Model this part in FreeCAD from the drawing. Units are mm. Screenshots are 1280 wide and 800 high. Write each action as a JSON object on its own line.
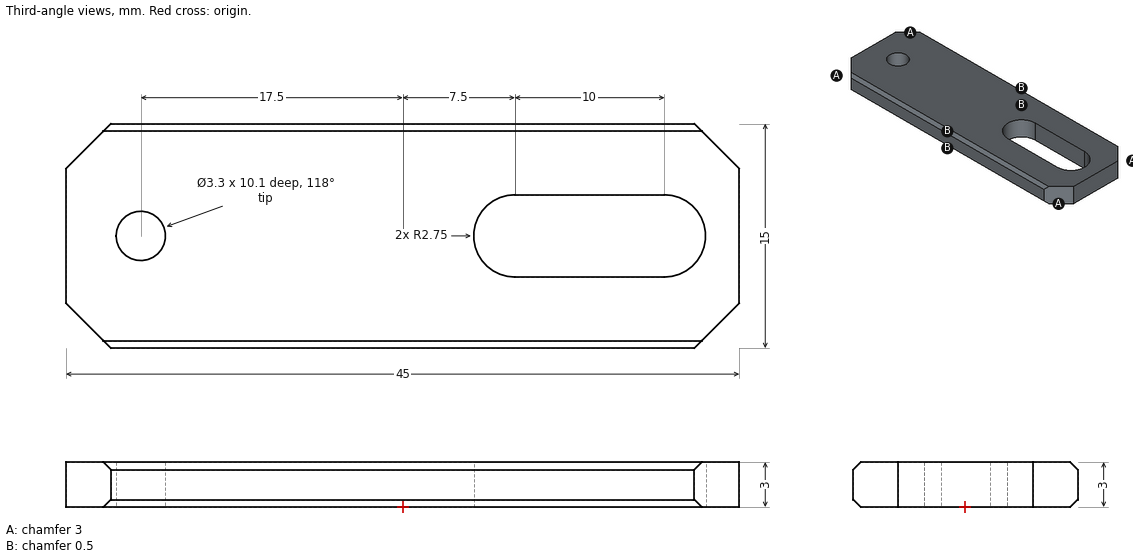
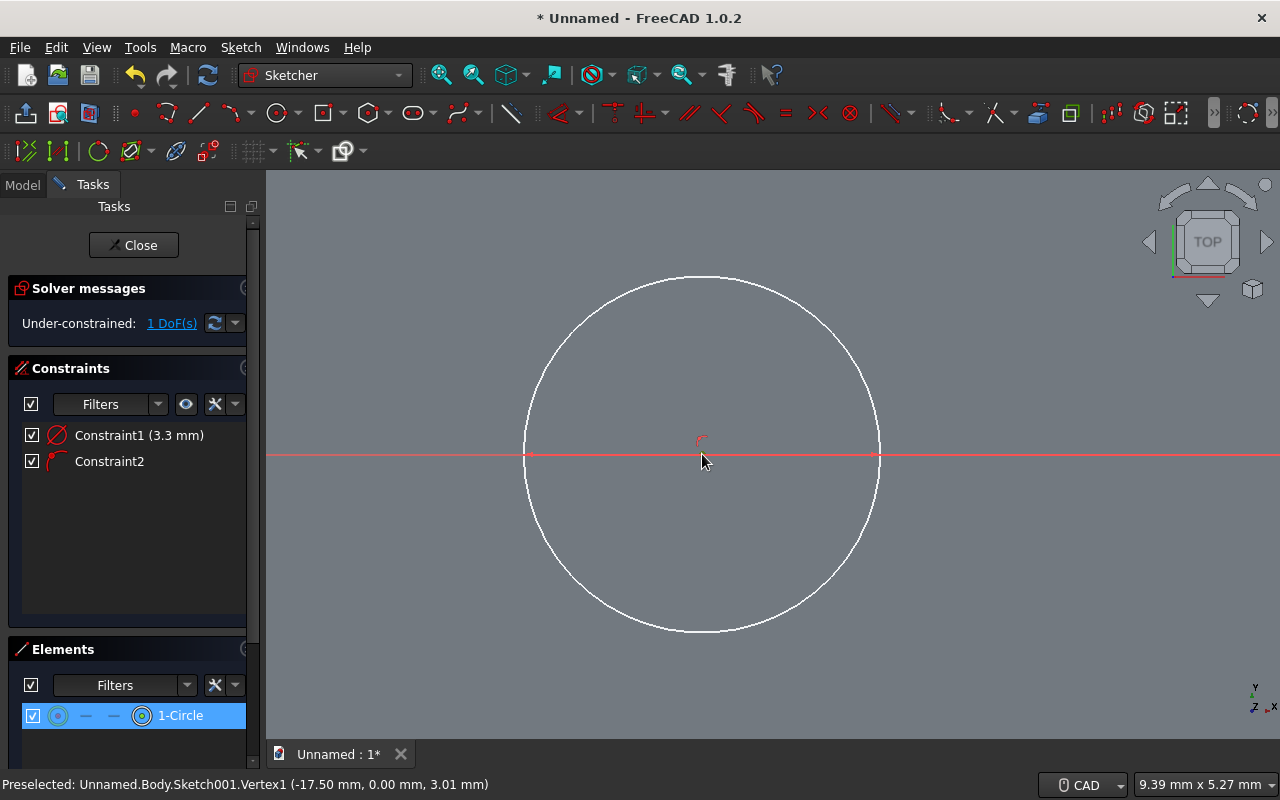
{"action": "key", "text": "l"}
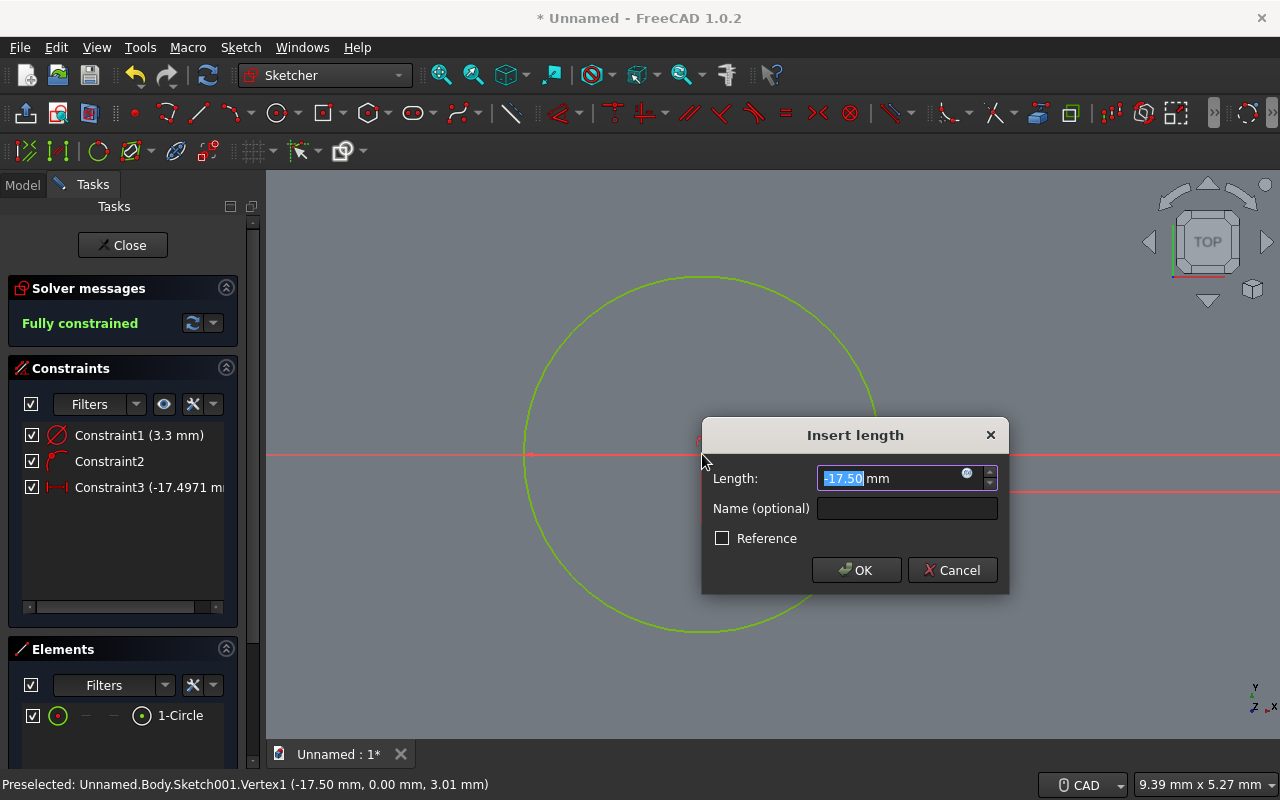
{"action": "type", "text": "-17.5"}
{"action": "key", "text": "Return"}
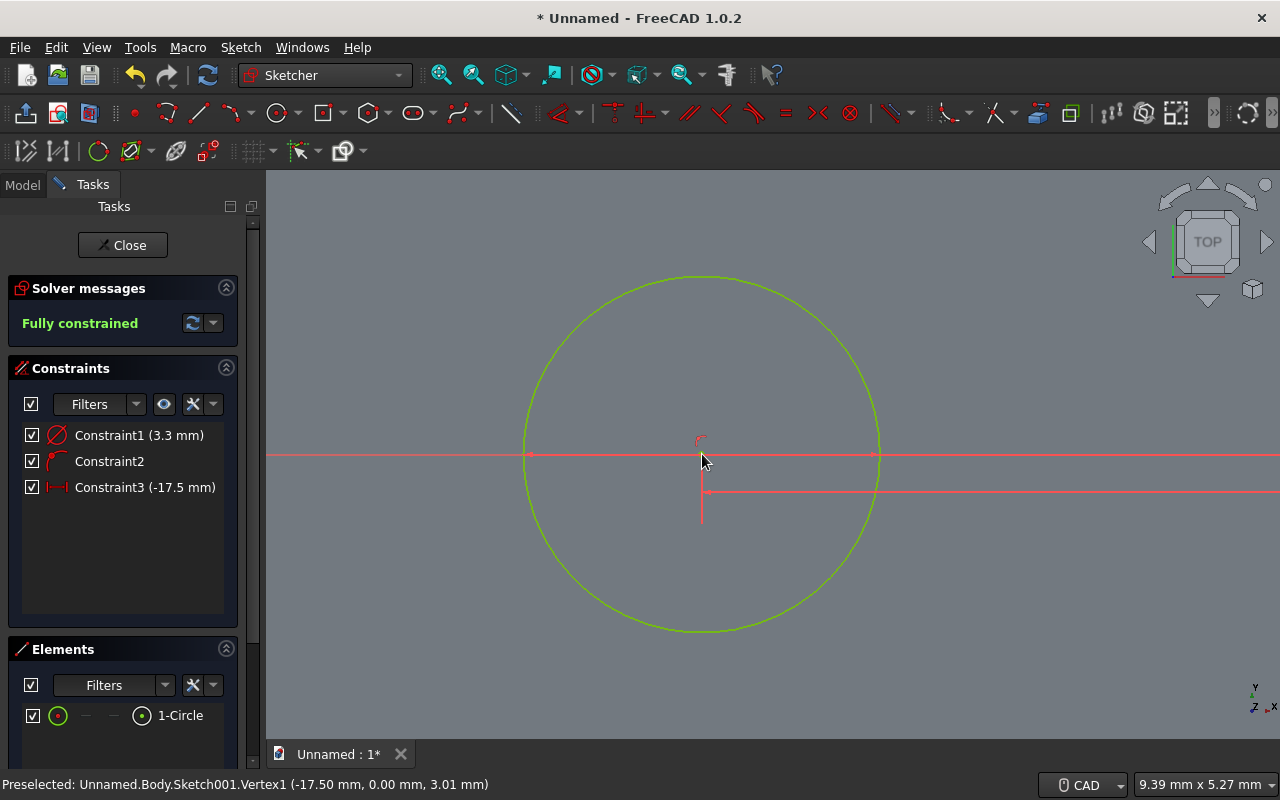
{"action": "left_click", "coordinate": [123, 245]}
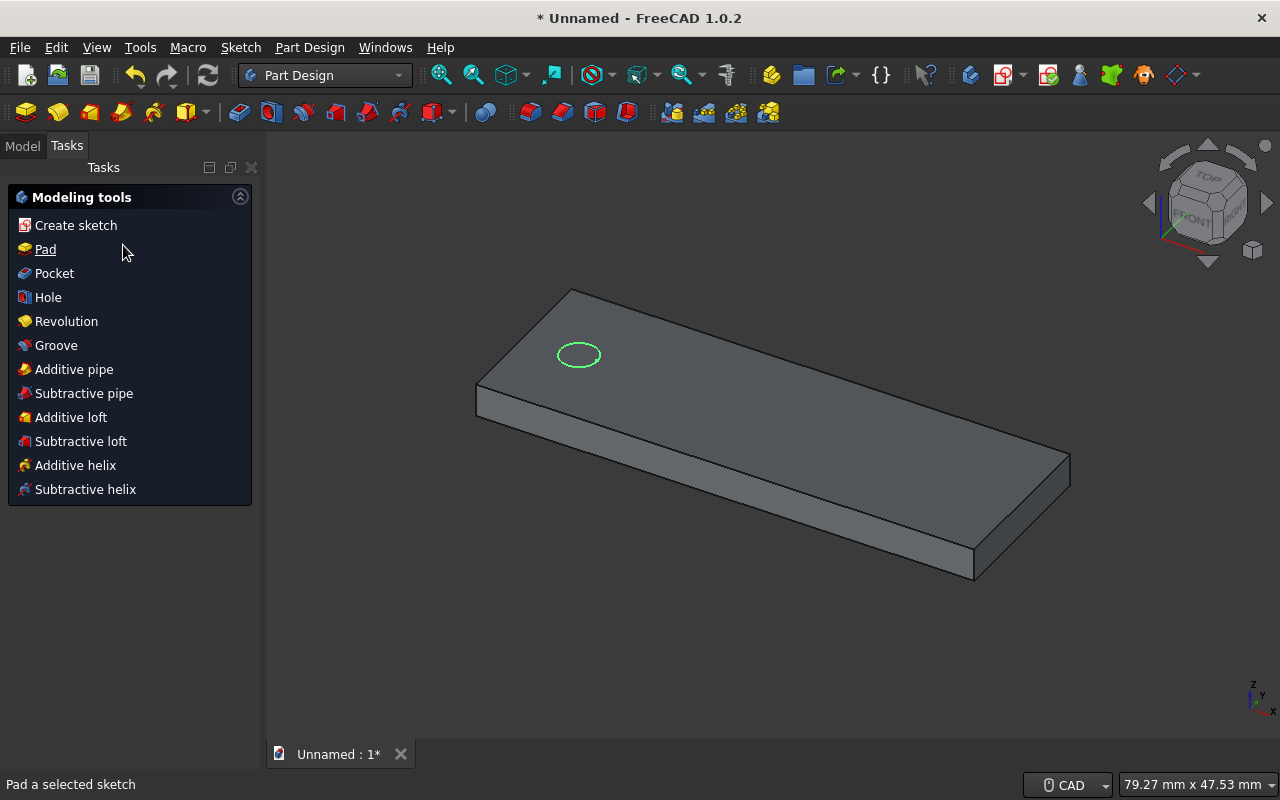
{"action": "left_click", "coordinate": [272, 112]}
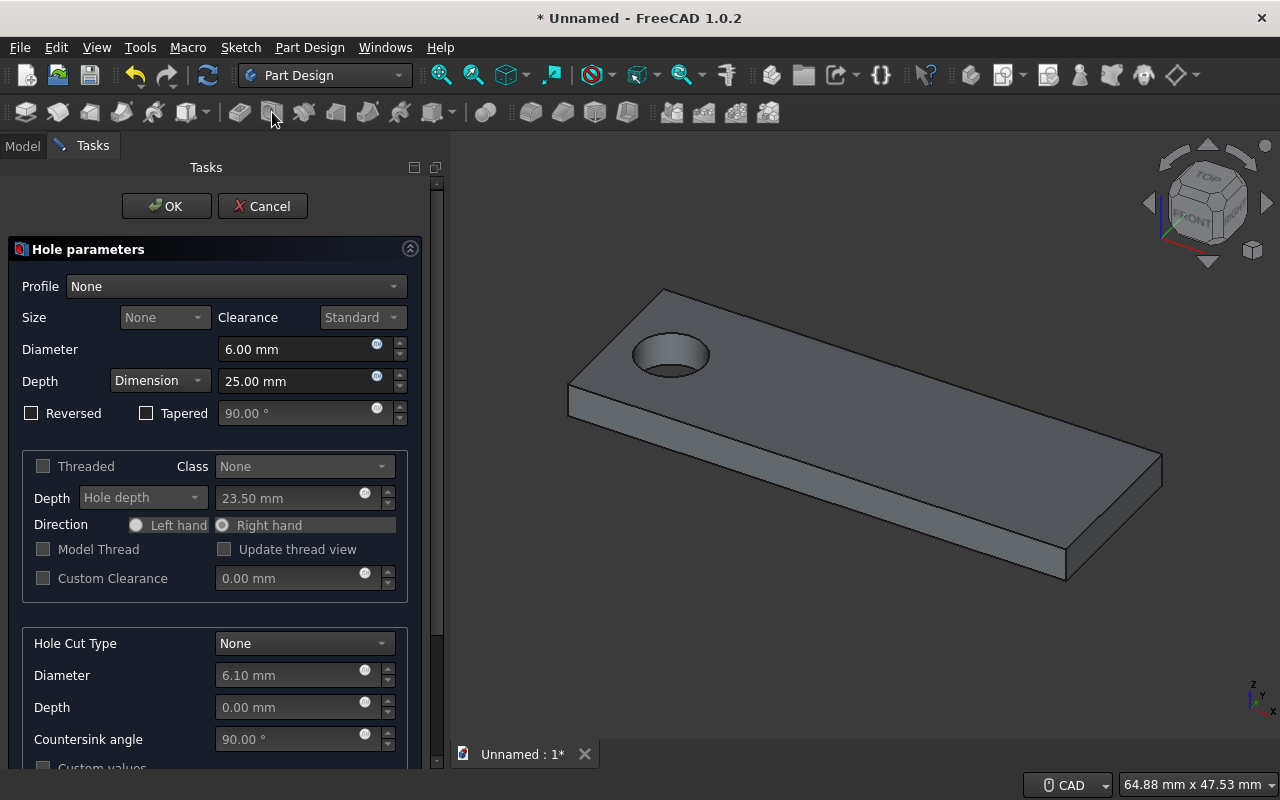
{"action": "triple_click", "coordinate": [305, 349]}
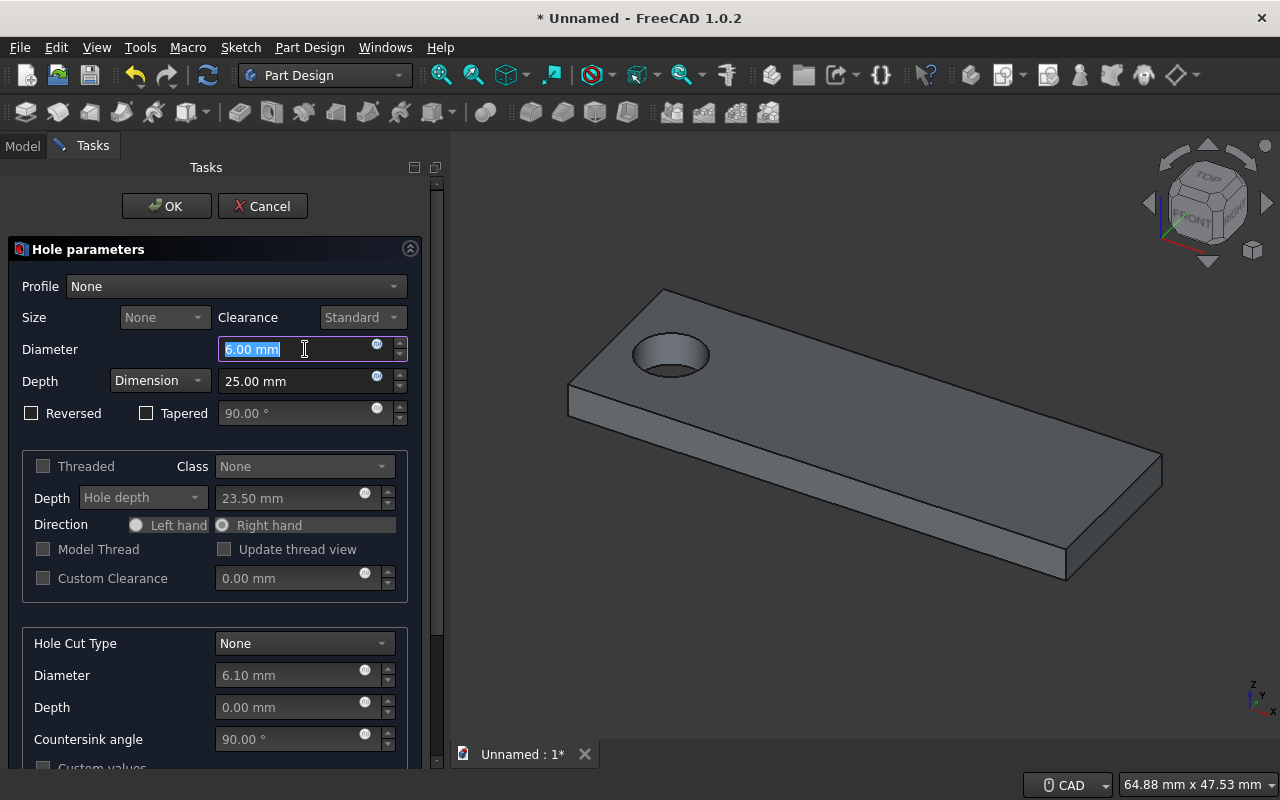
{"action": "type", "text": "3.3"}
{"action": "key", "text": "Tab"}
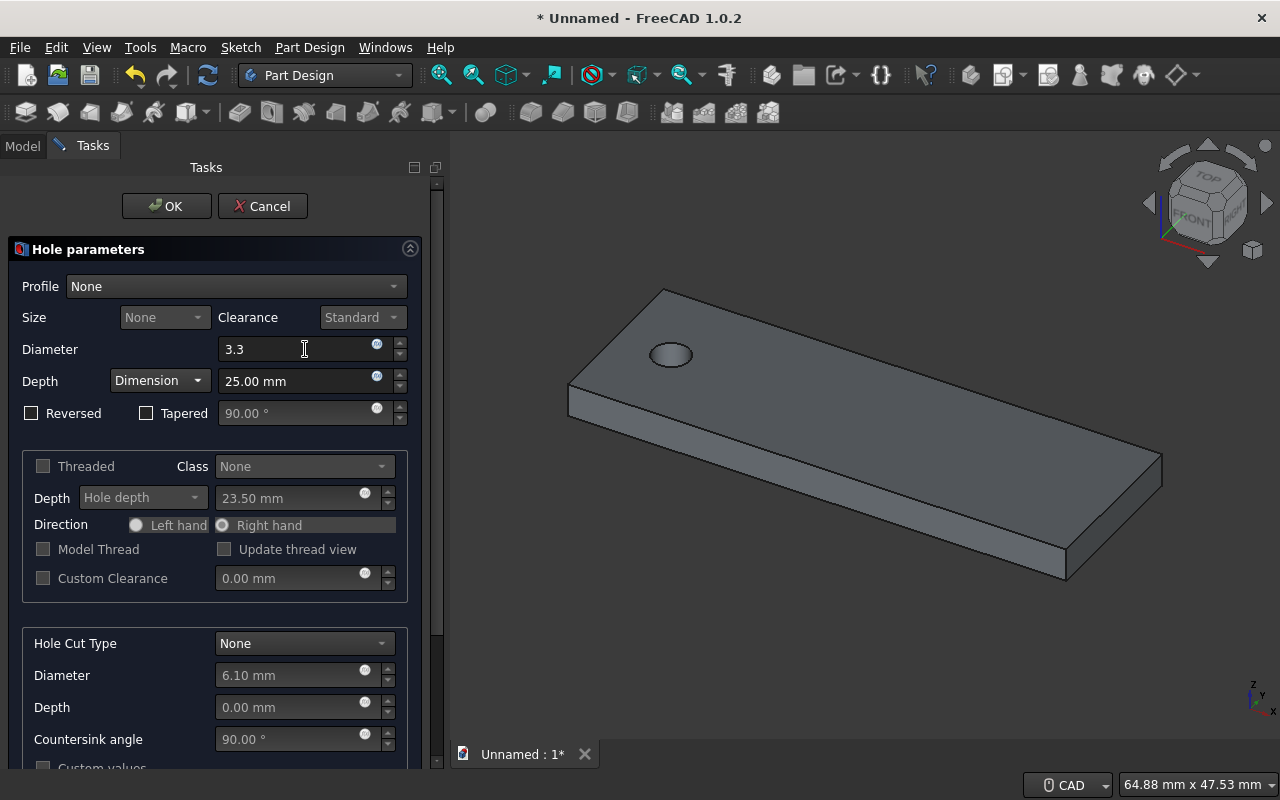
{"action": "triple_click", "coordinate": [305, 381]}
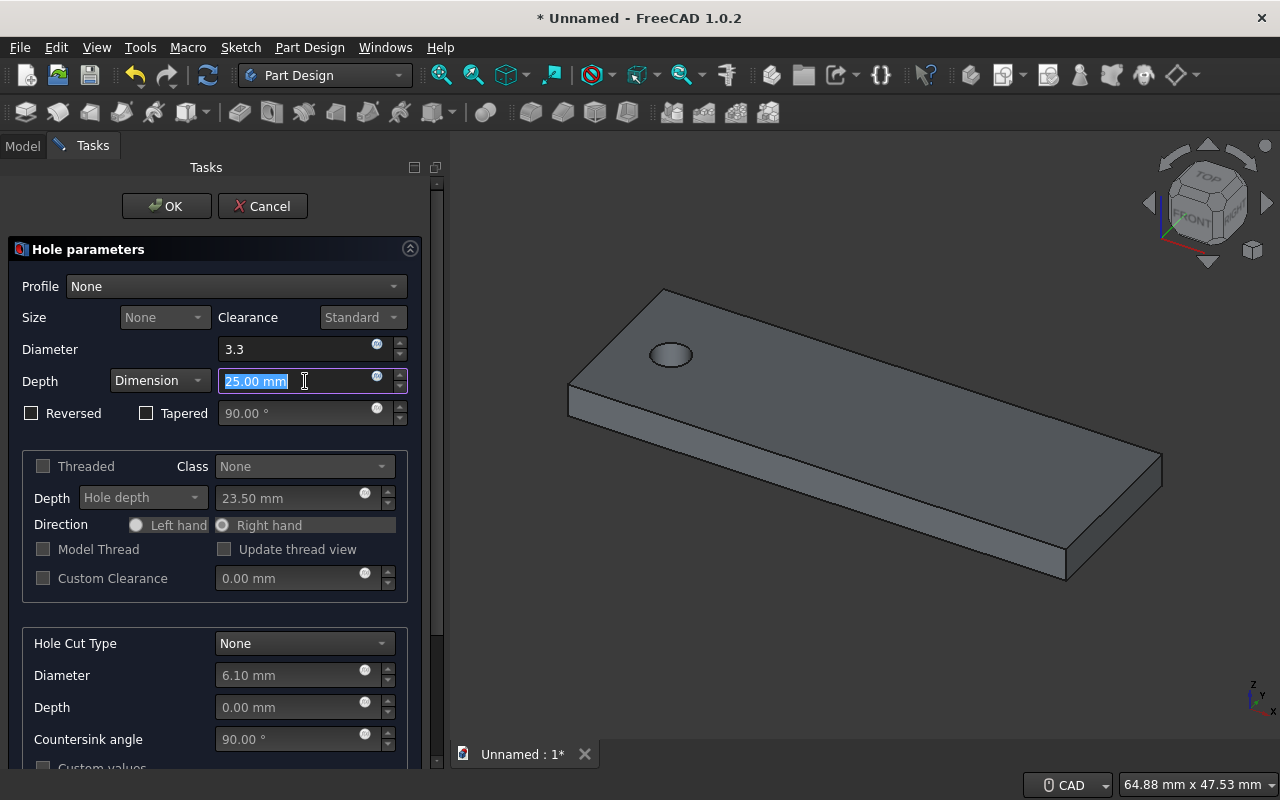
{"action": "type", "text": "10.1"}
{"action": "key", "text": "Tab"}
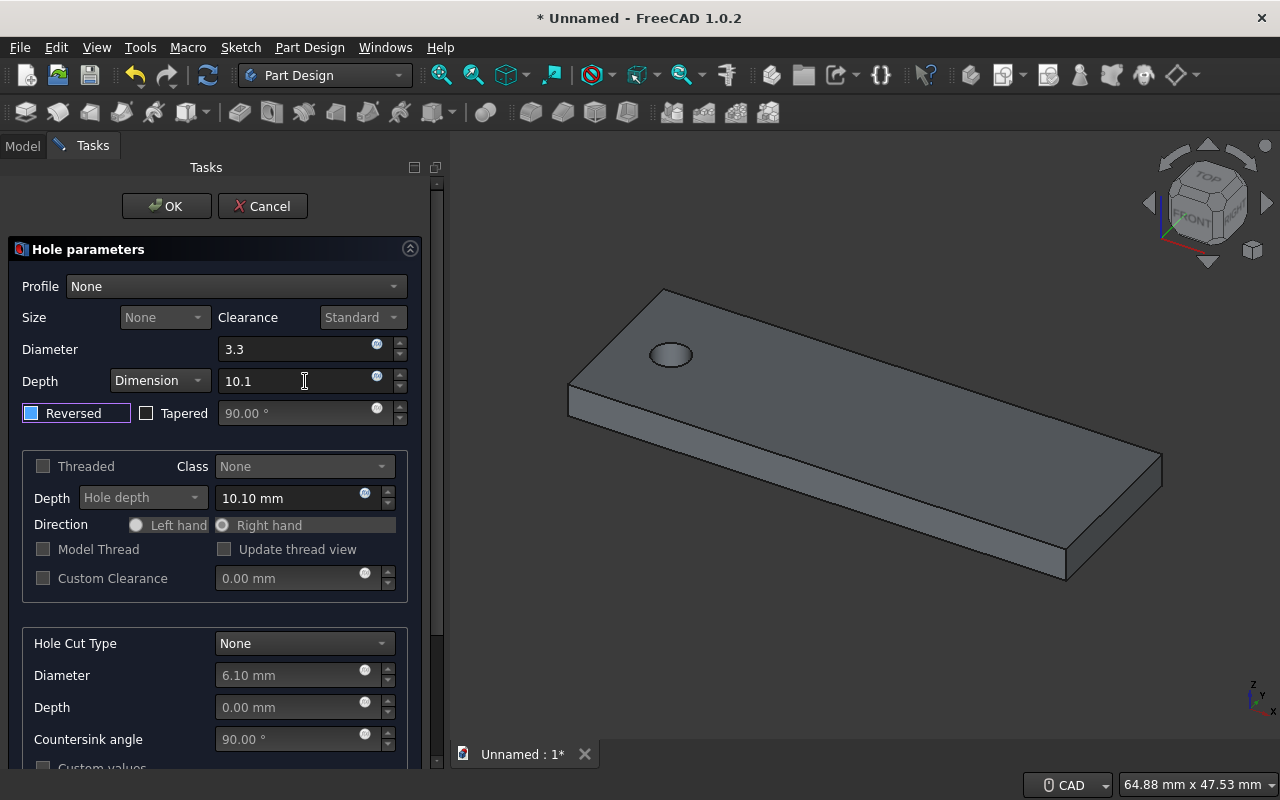
{"action": "left_click", "coordinate": [167, 206]}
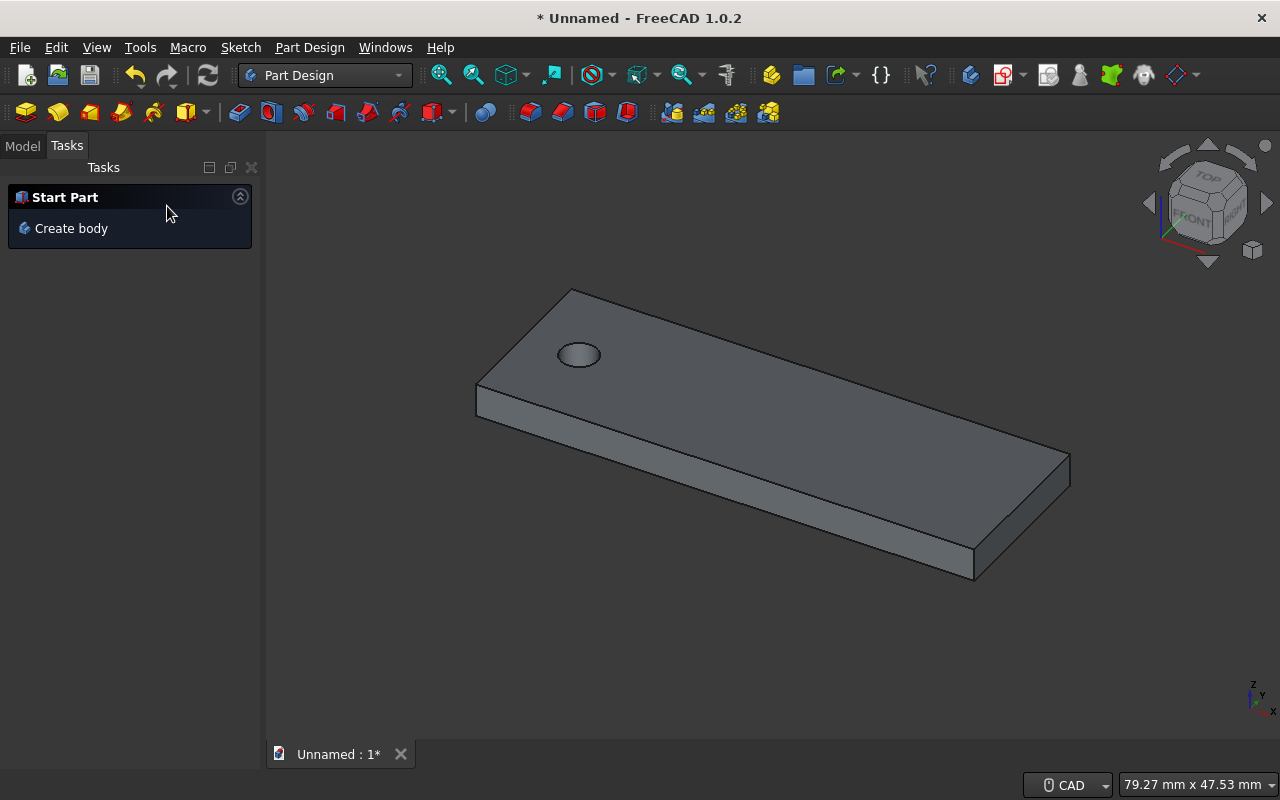
{"action": "left_click", "coordinate": [915, 465]}